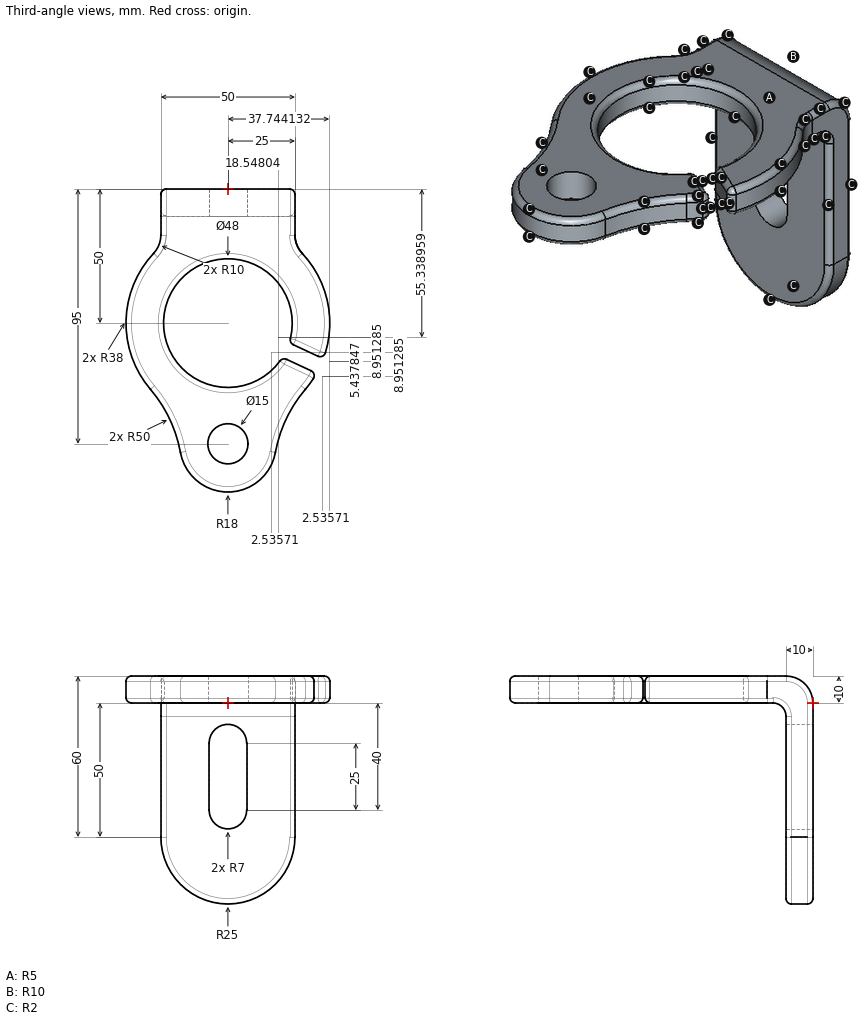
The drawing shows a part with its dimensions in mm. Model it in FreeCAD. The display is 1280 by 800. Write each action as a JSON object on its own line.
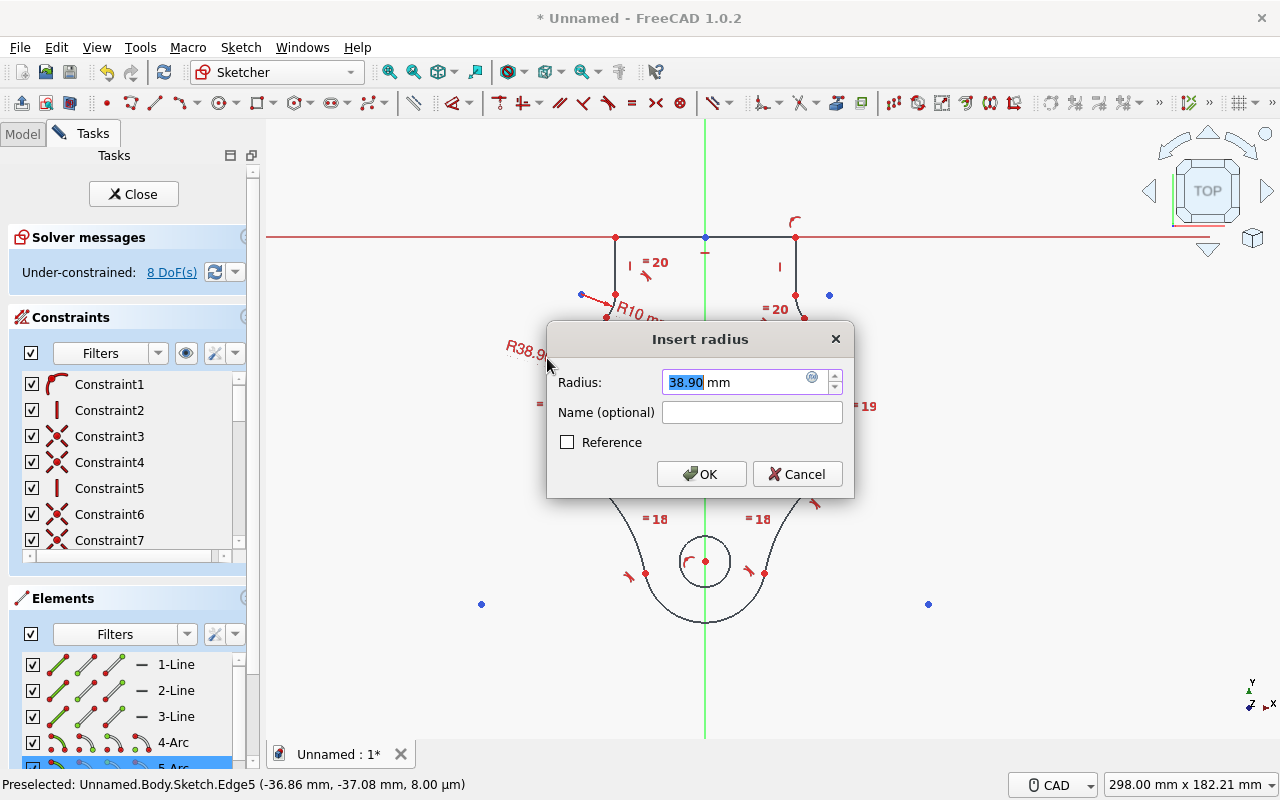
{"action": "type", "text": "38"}
{"action": "key", "text": "Return"}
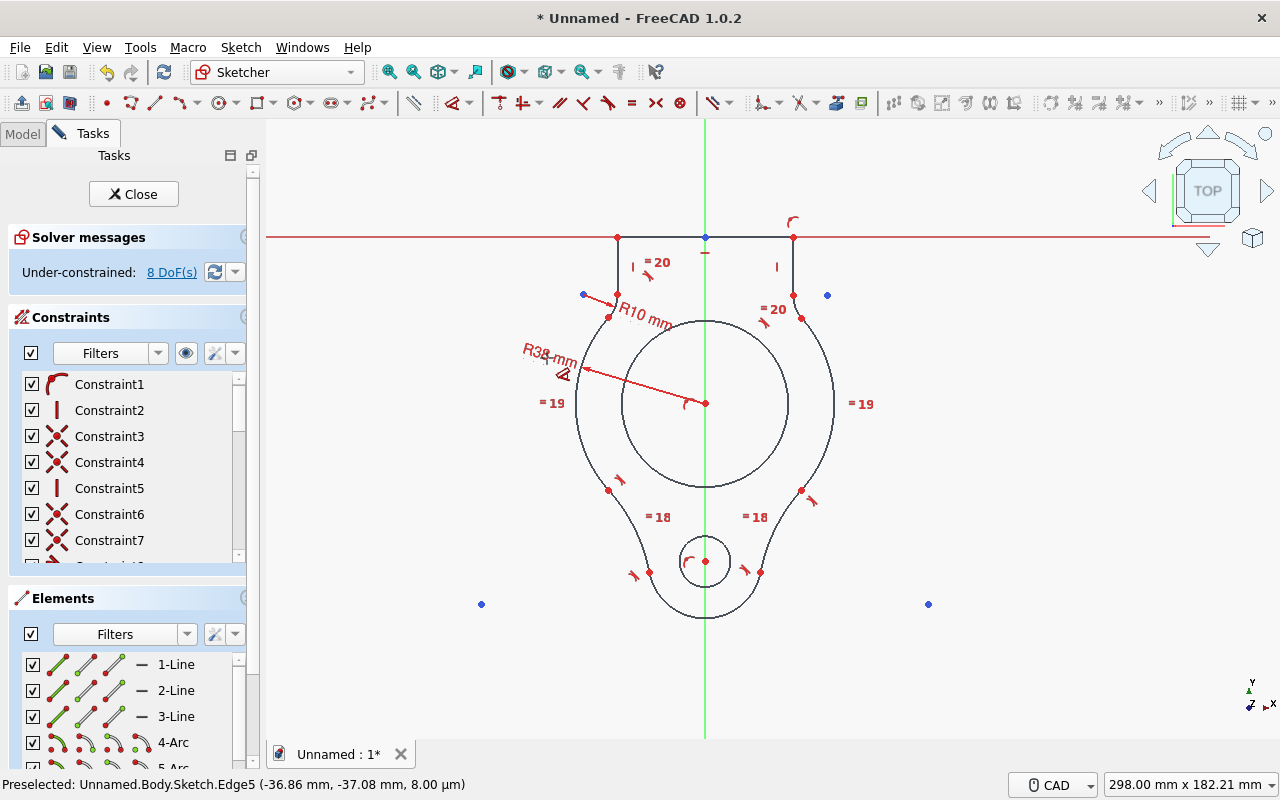
{"action": "left_click", "coordinate": [642, 546]}
{"action": "left_click", "coordinate": [672, 535]}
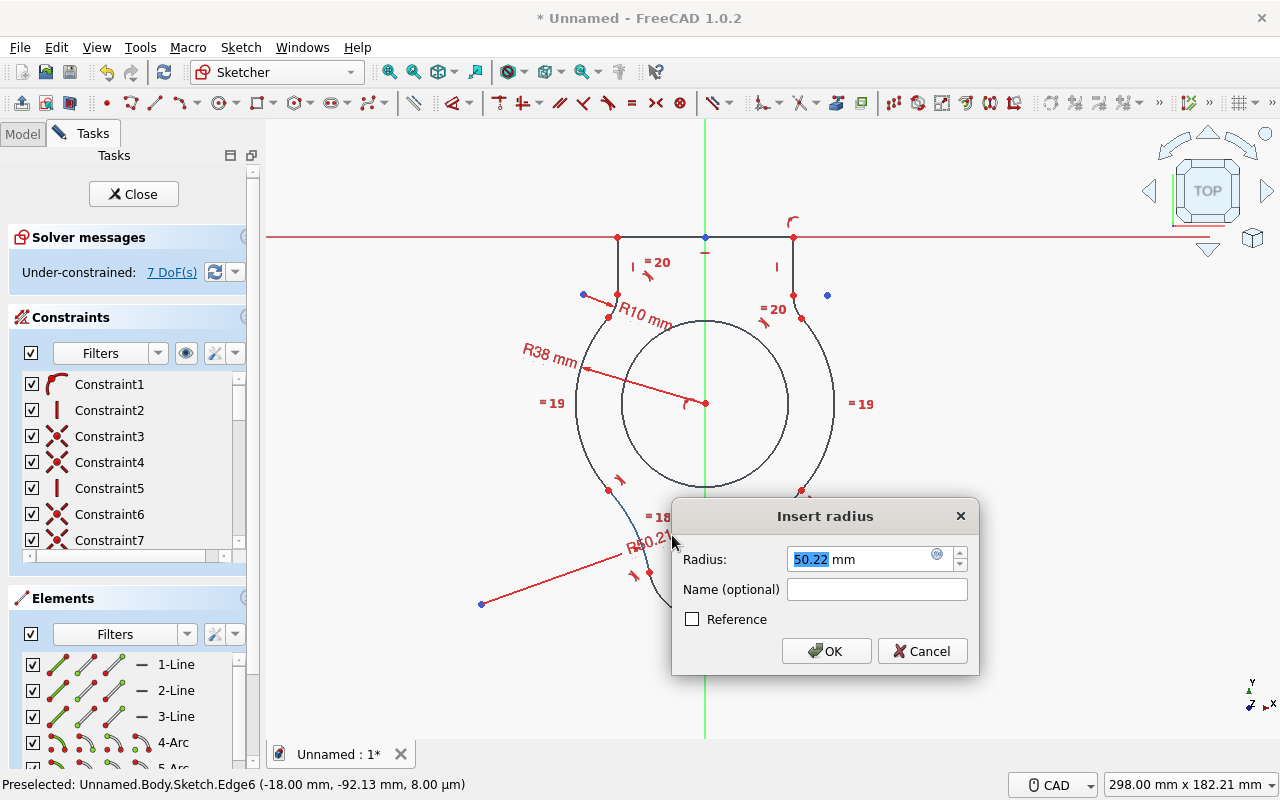
{"action": "type", "text": "50"}
{"action": "key", "text": "Return"}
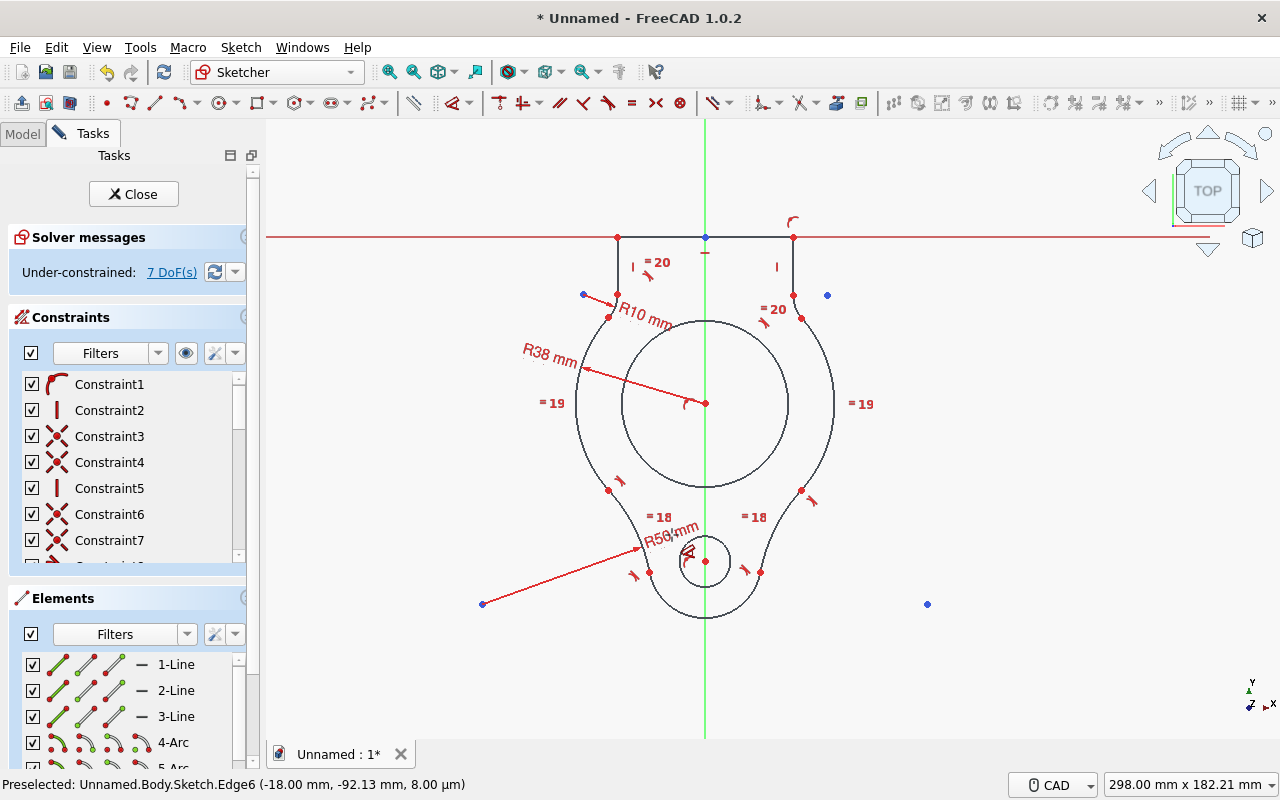
{"action": "left_click", "coordinate": [675, 610]}
{"action": "left_click", "coordinate": [658, 637]}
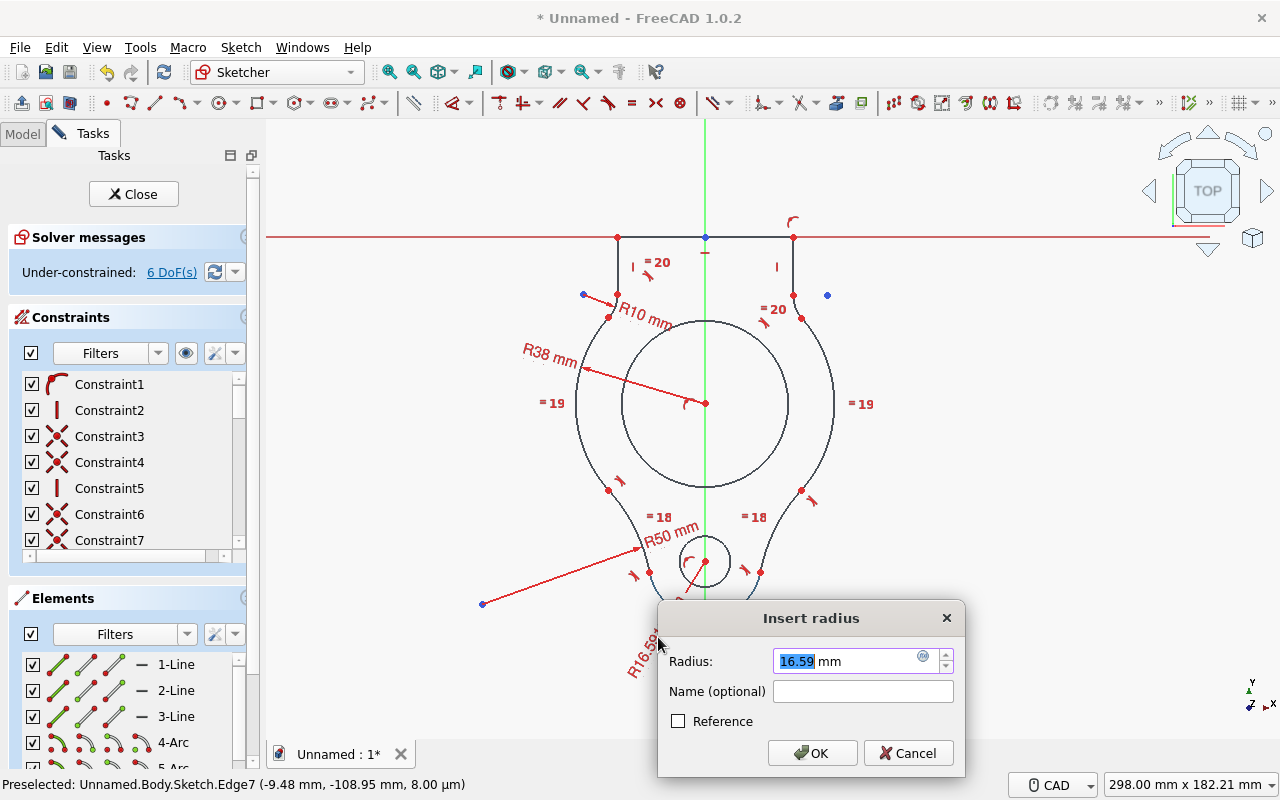
{"action": "type", "text": "18"}
{"action": "key", "text": "Return"}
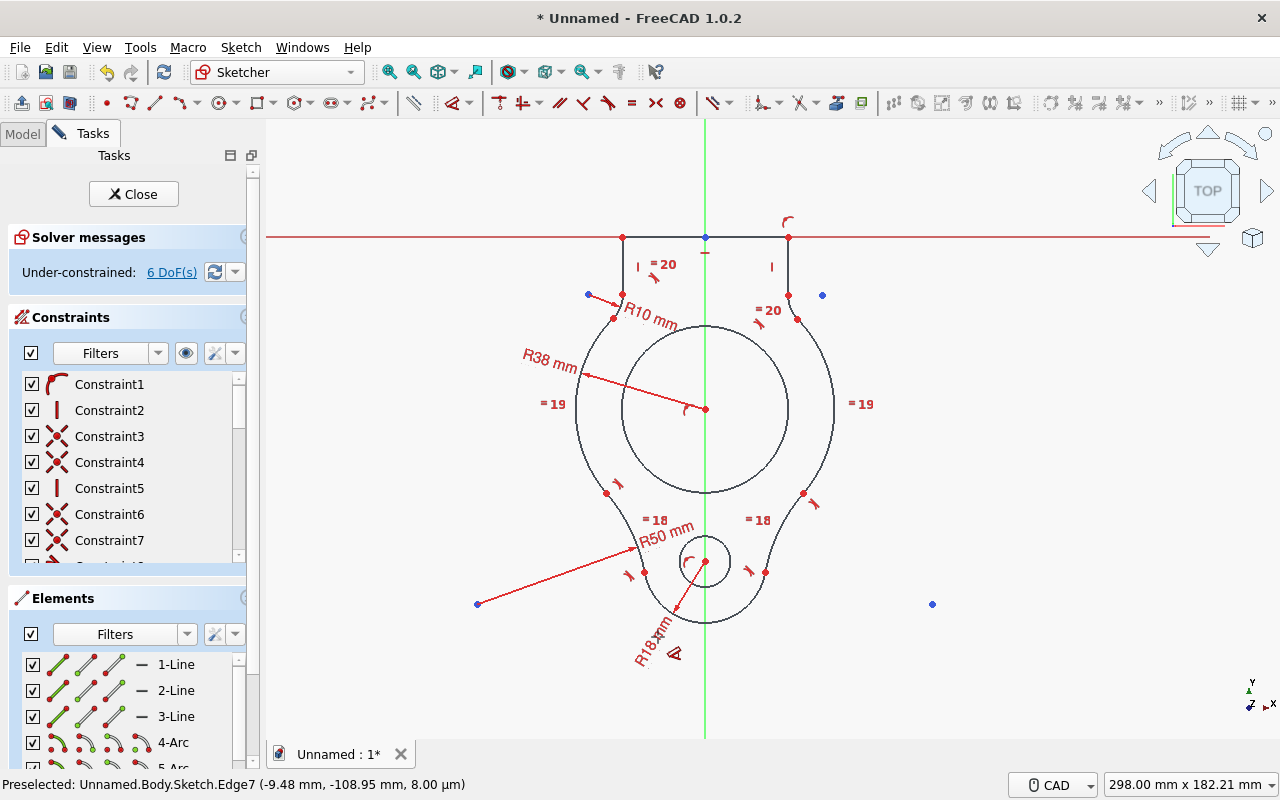
{"action": "left_click", "coordinate": [723, 544]}
{"action": "left_click", "coordinate": [746, 522]}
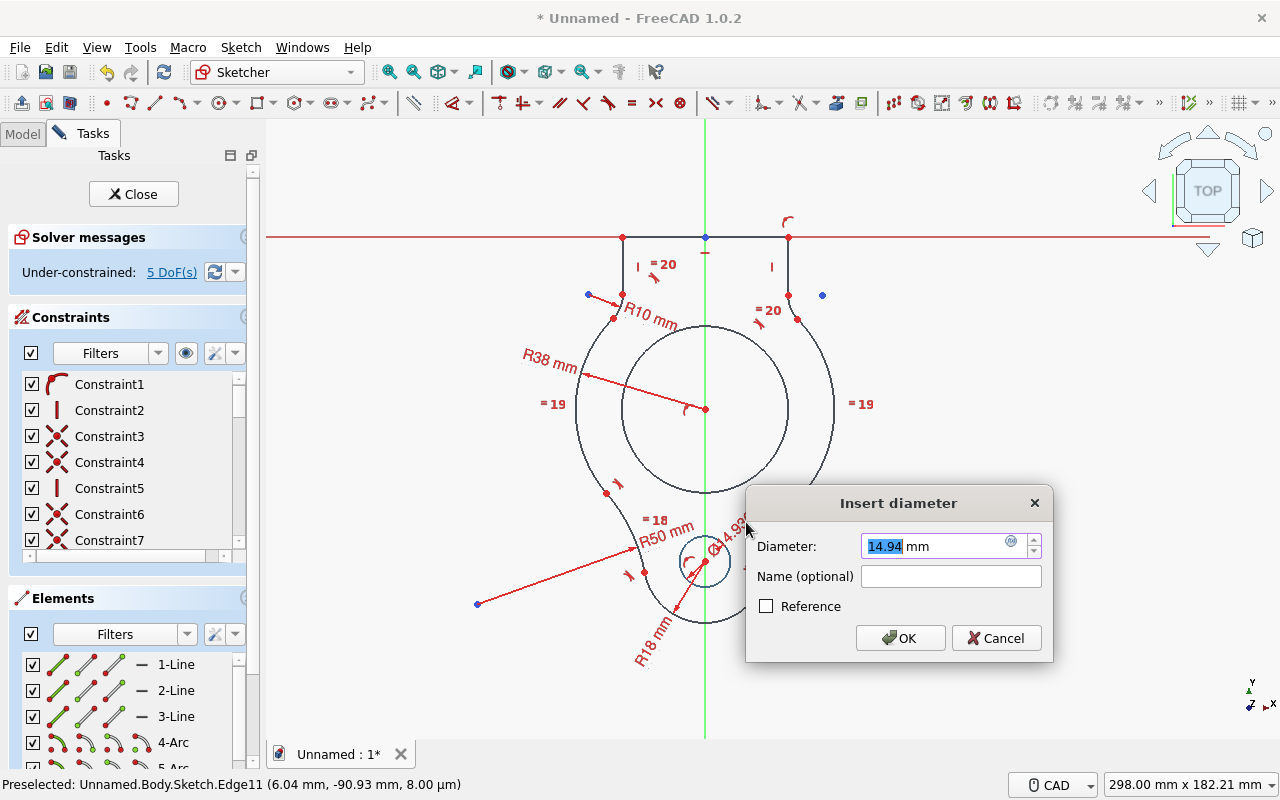
{"action": "type", "text": "15"}
{"action": "key", "text": "Return"}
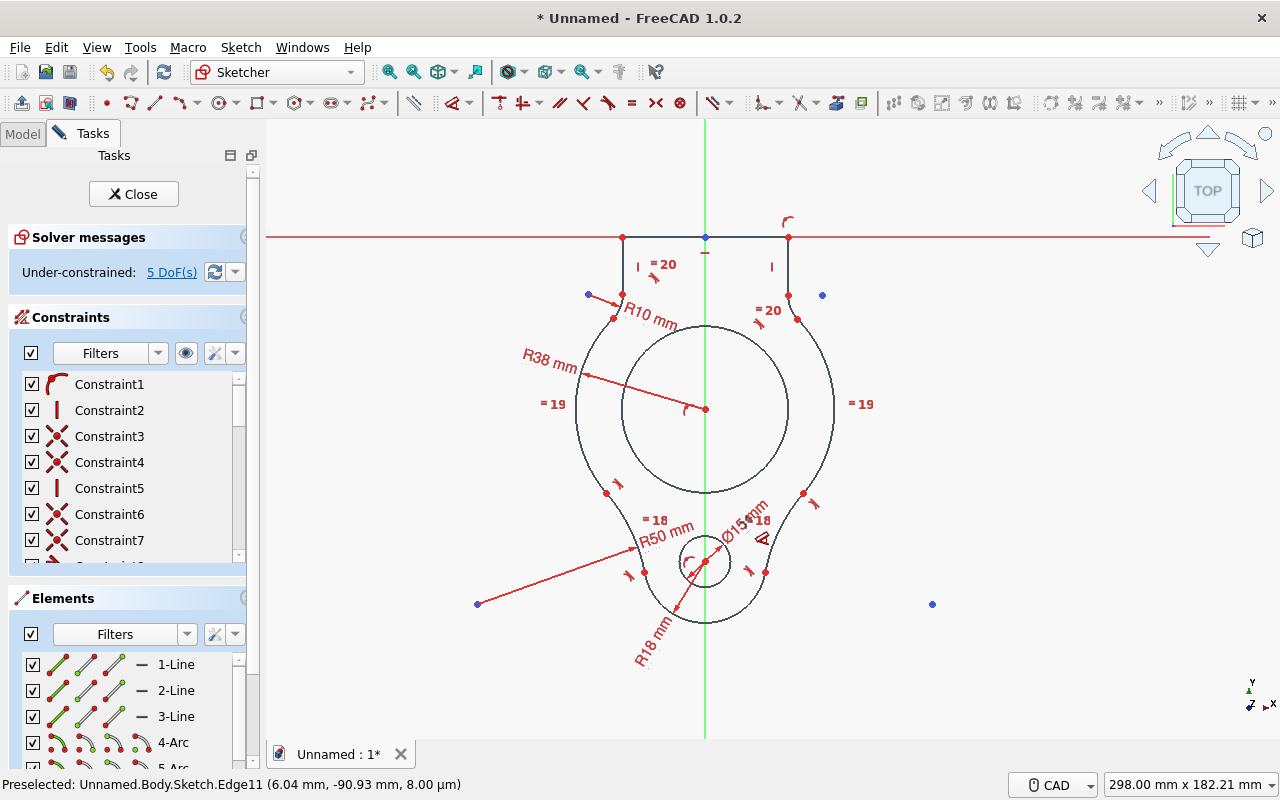
{"action": "left_click", "coordinate": [764, 350]}
{"action": "left_click", "coordinate": [787, 327]}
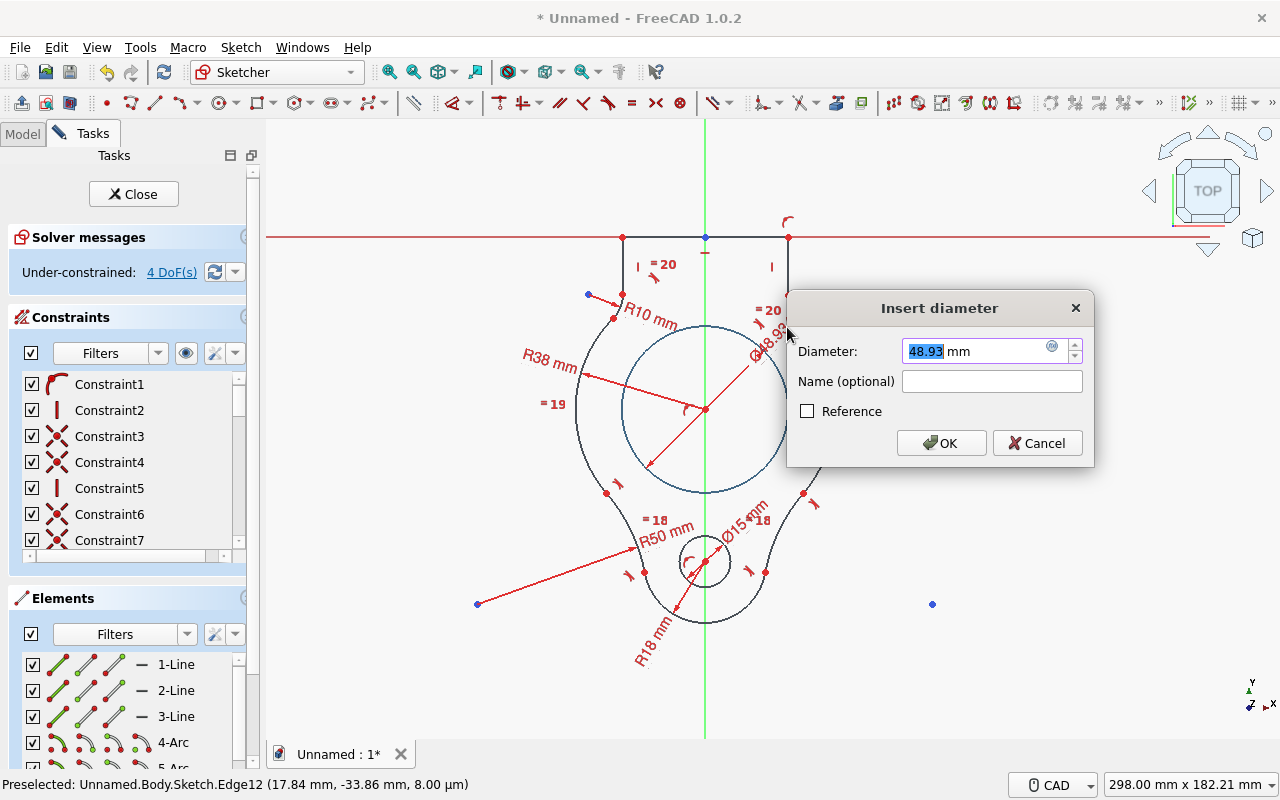
{"action": "type", "text": "48"}
{"action": "key", "text": "Return"}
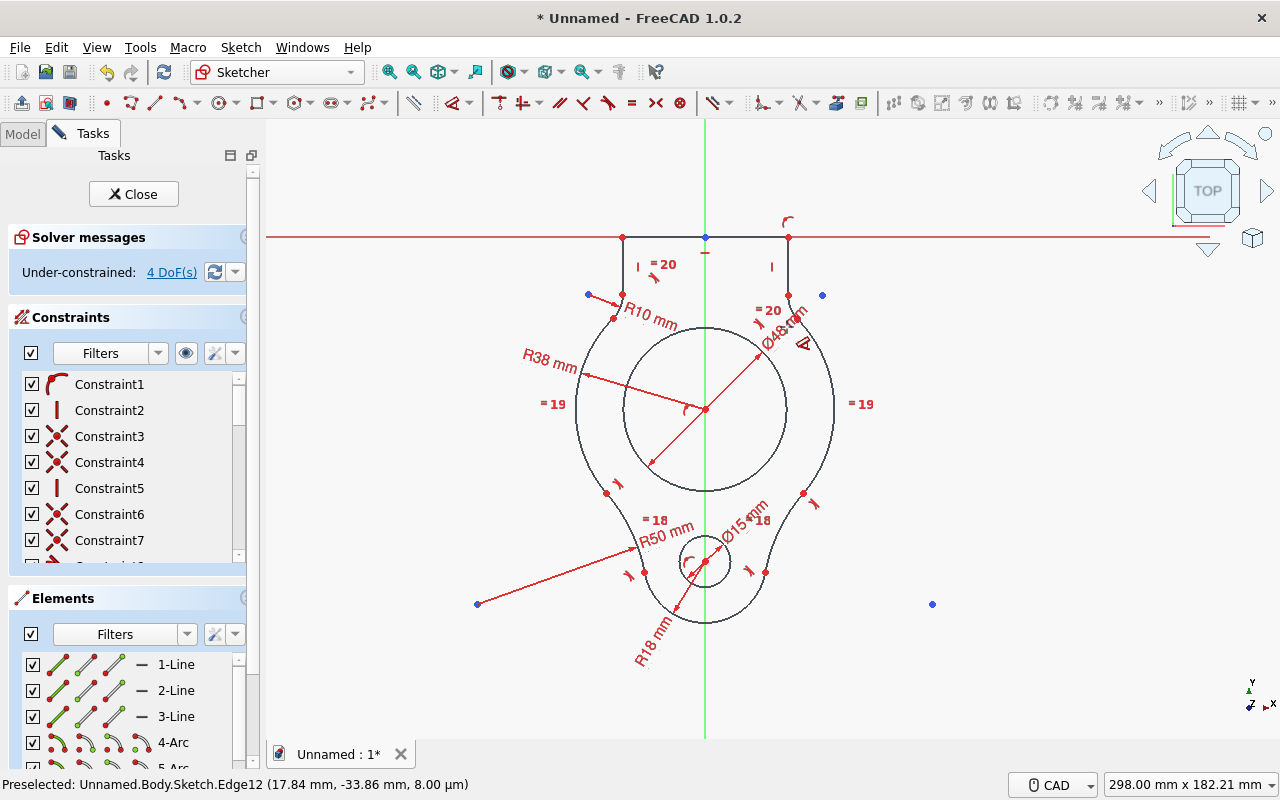
{"action": "left_click", "coordinate": [739, 237]}
{"action": "left_click", "coordinate": [668, 203]}